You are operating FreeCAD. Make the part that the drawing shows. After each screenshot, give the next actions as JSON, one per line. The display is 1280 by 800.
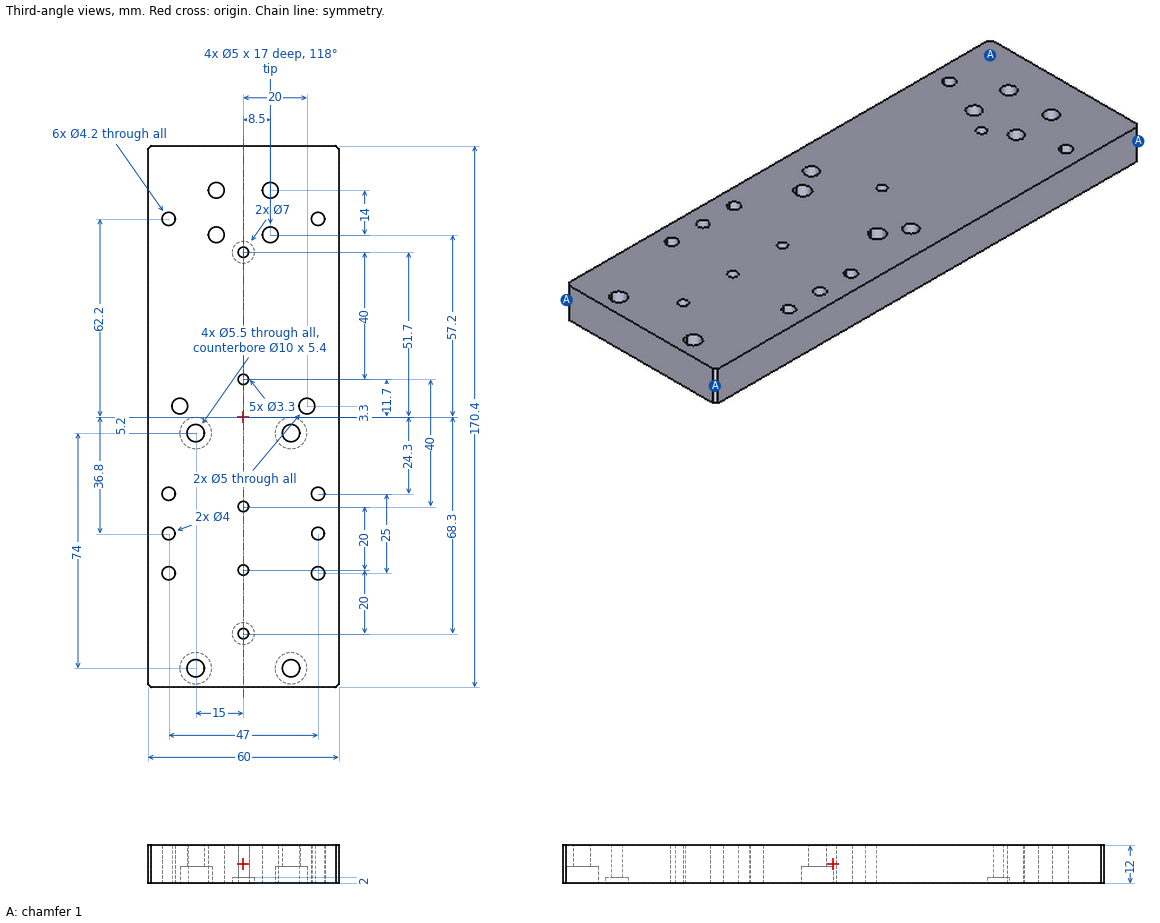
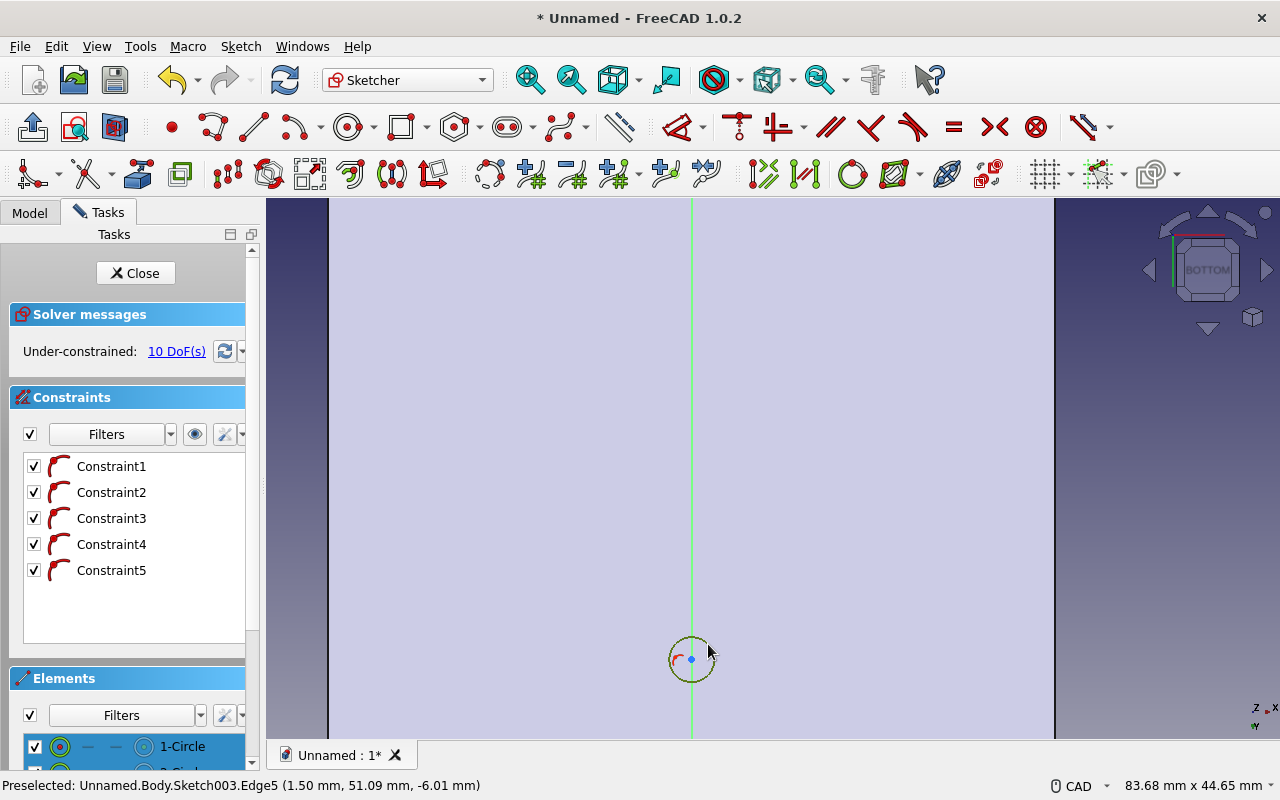
{"action": "left_click", "coordinate": [954, 128]}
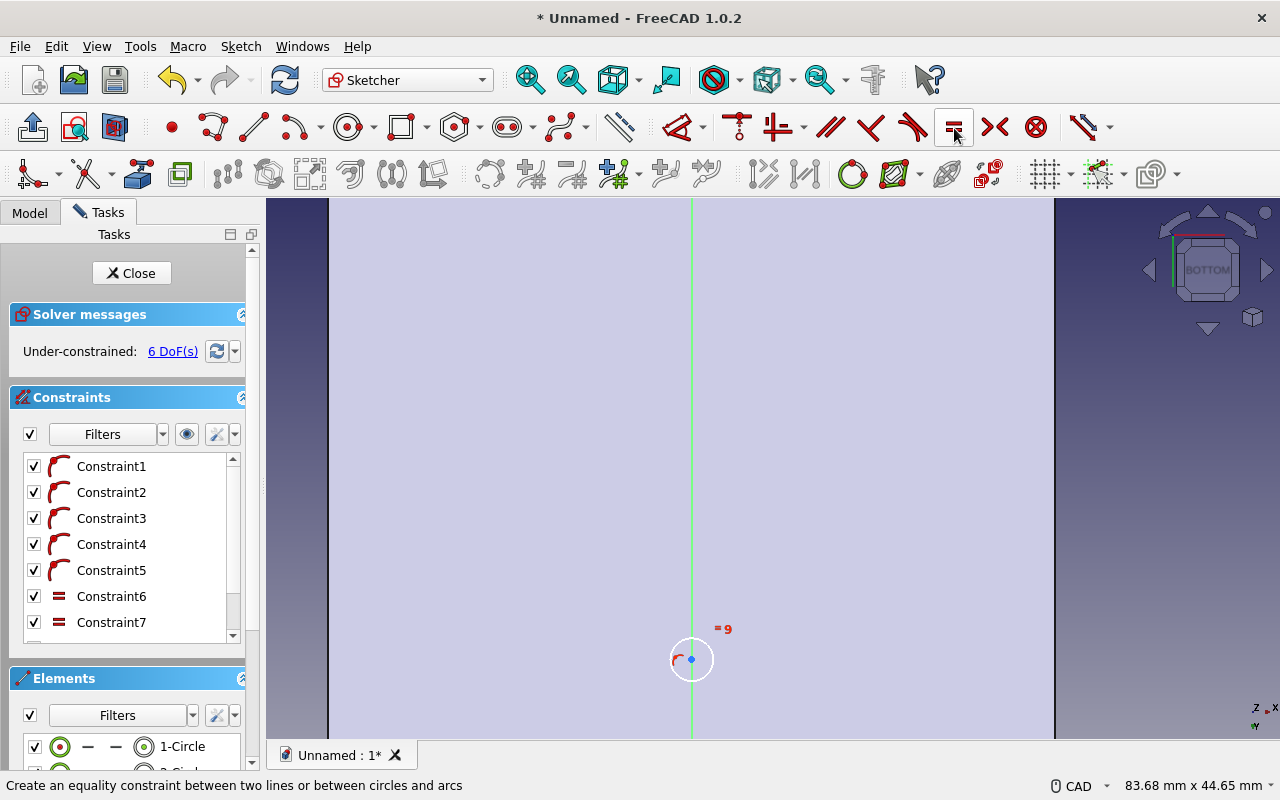
{"action": "left_click", "coordinate": [676, 128]}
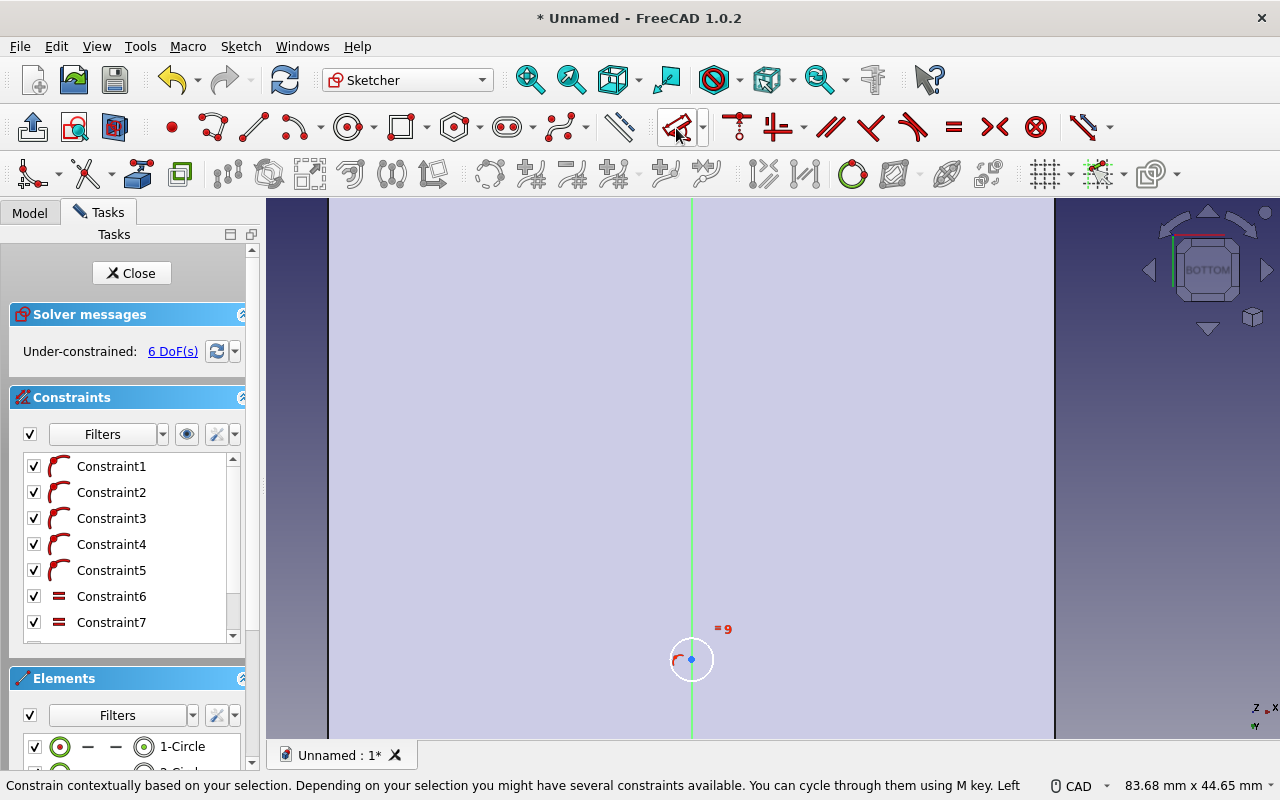
{"action": "scroll", "coordinate": [709, 646], "scroll_direction": "down", "scroll_amount": 7}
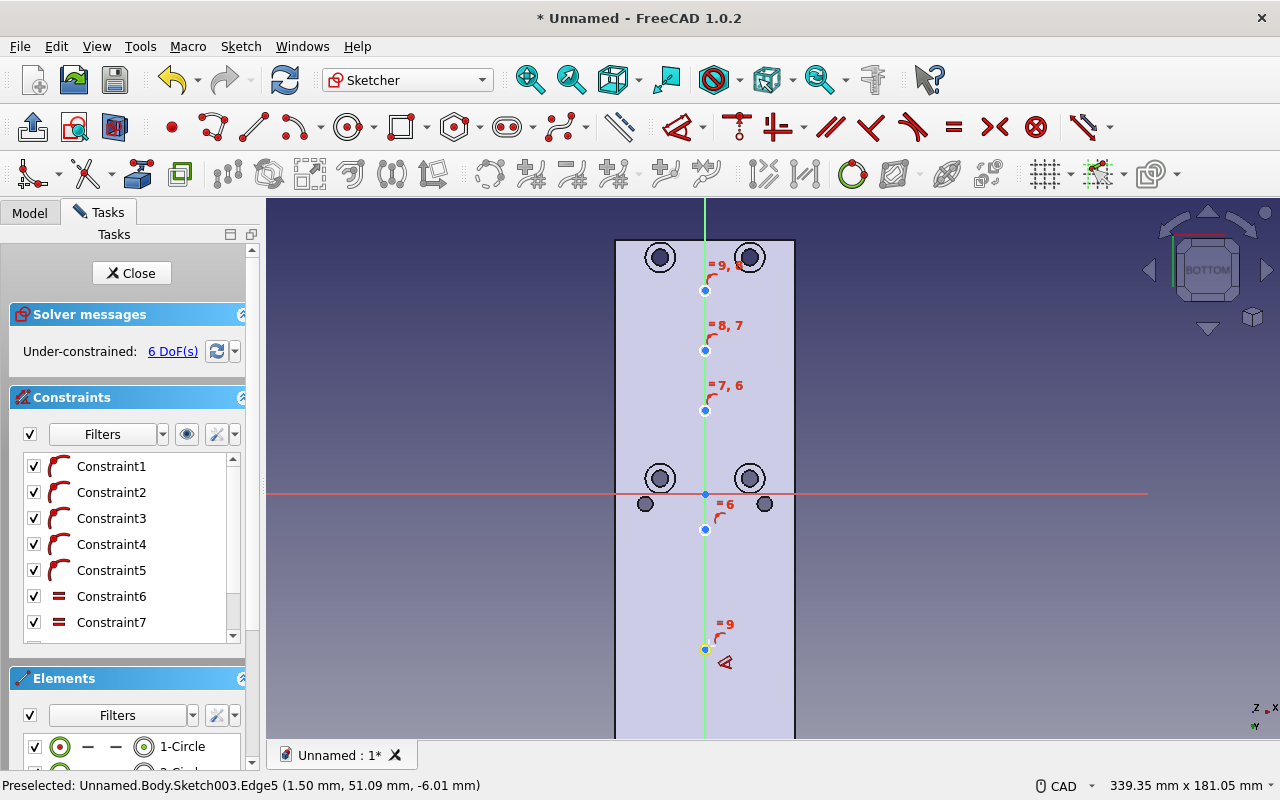
{"action": "scroll", "coordinate": [709, 526], "scroll_direction": "up", "scroll_amount": 7}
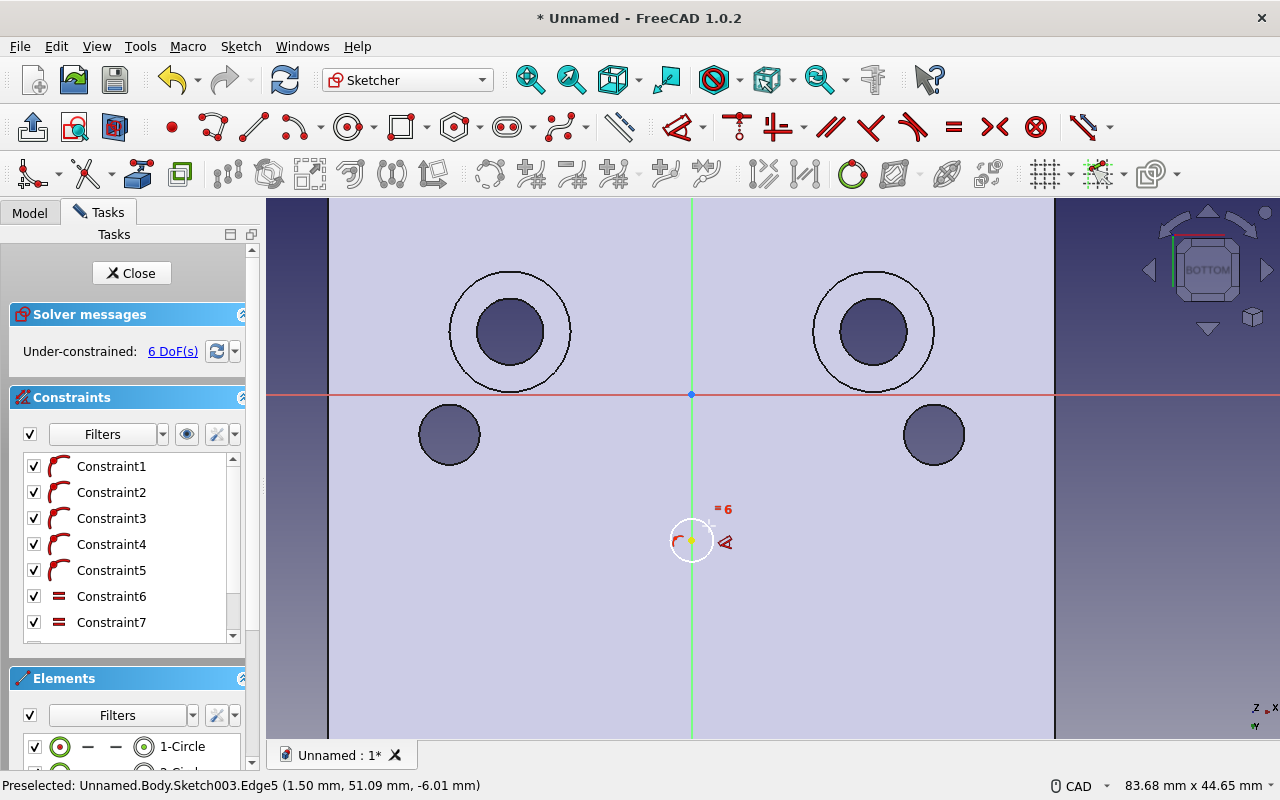
{"action": "left_click", "coordinate": [707, 525]}
{"action": "left_click", "coordinate": [729, 502]}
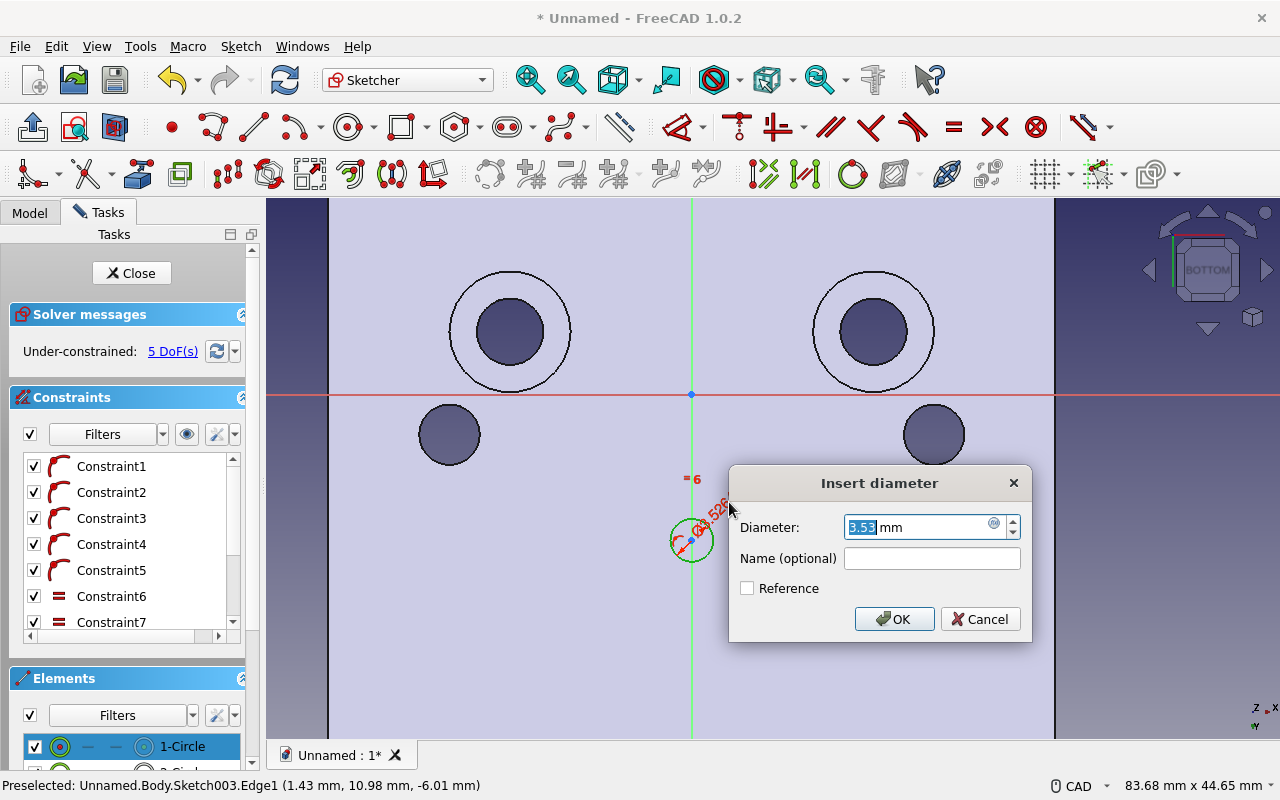
{"action": "type", "text": "3.3"}
{"action": "key", "text": "Return"}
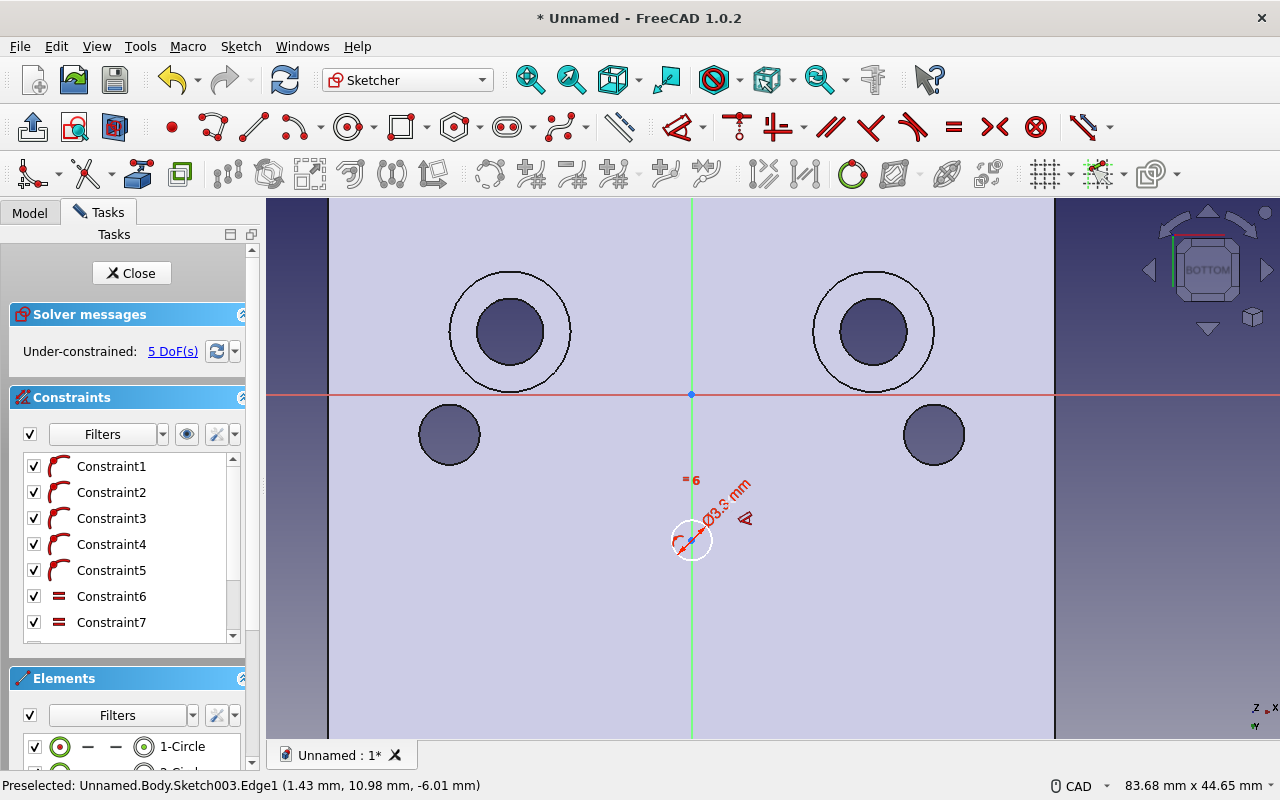
{"action": "scroll", "coordinate": [709, 526], "scroll_direction": "down", "scroll_amount": 7}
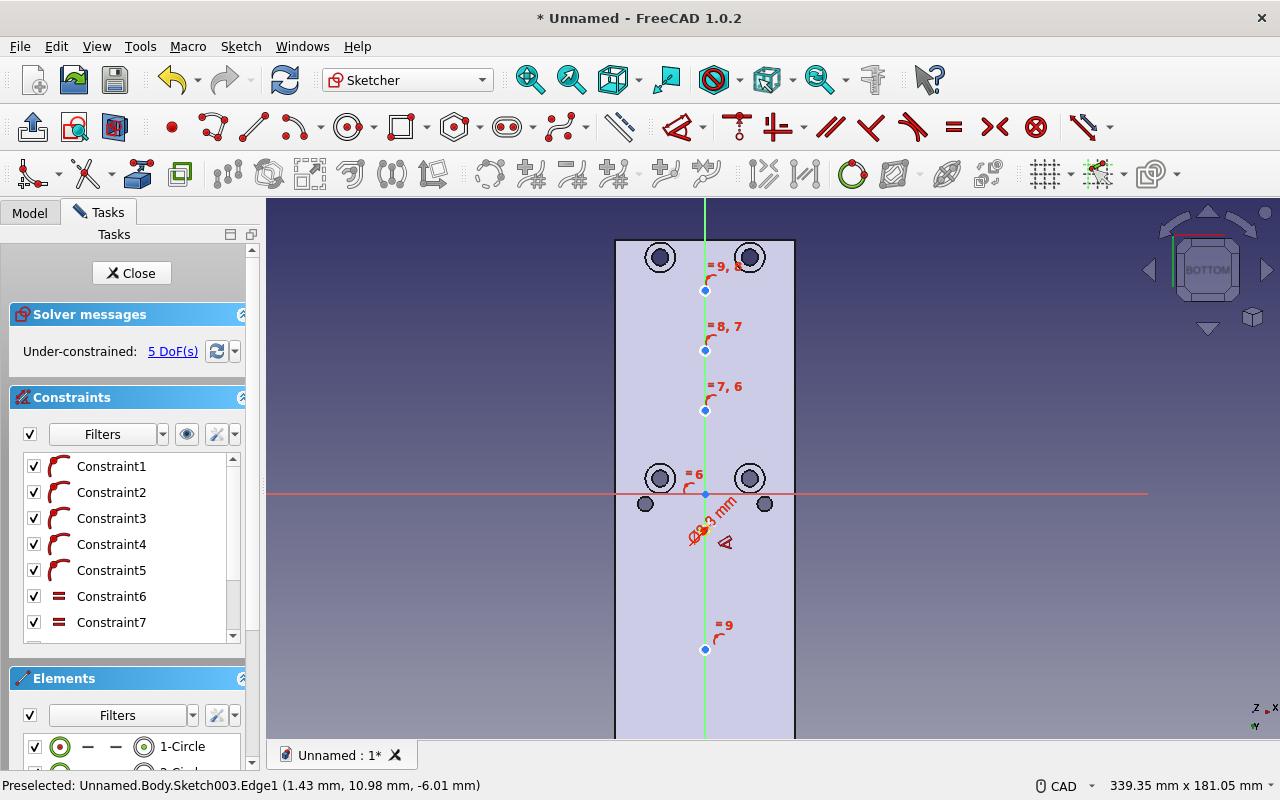
{"action": "left_click", "coordinate": [705, 530]}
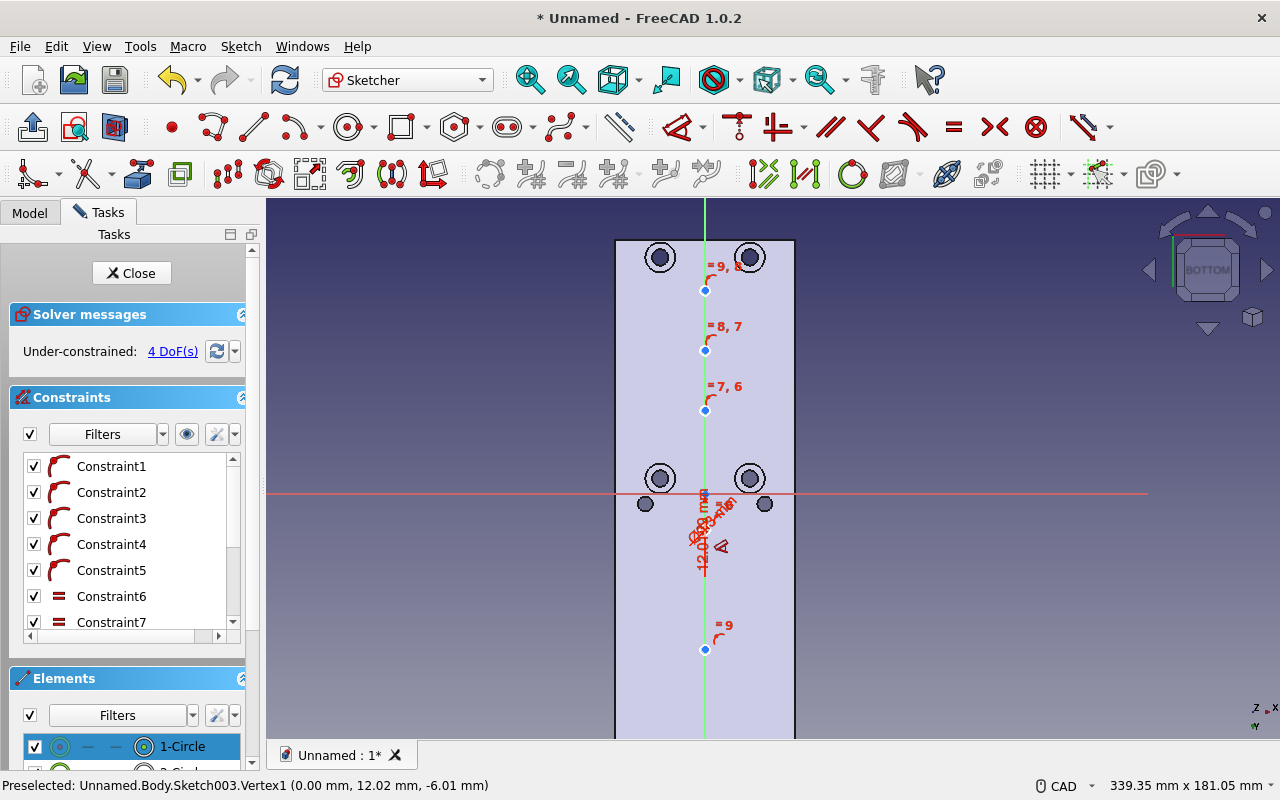
{"action": "left_click", "coordinate": [705, 411]}
{"action": "left_click", "coordinate": [739, 470]}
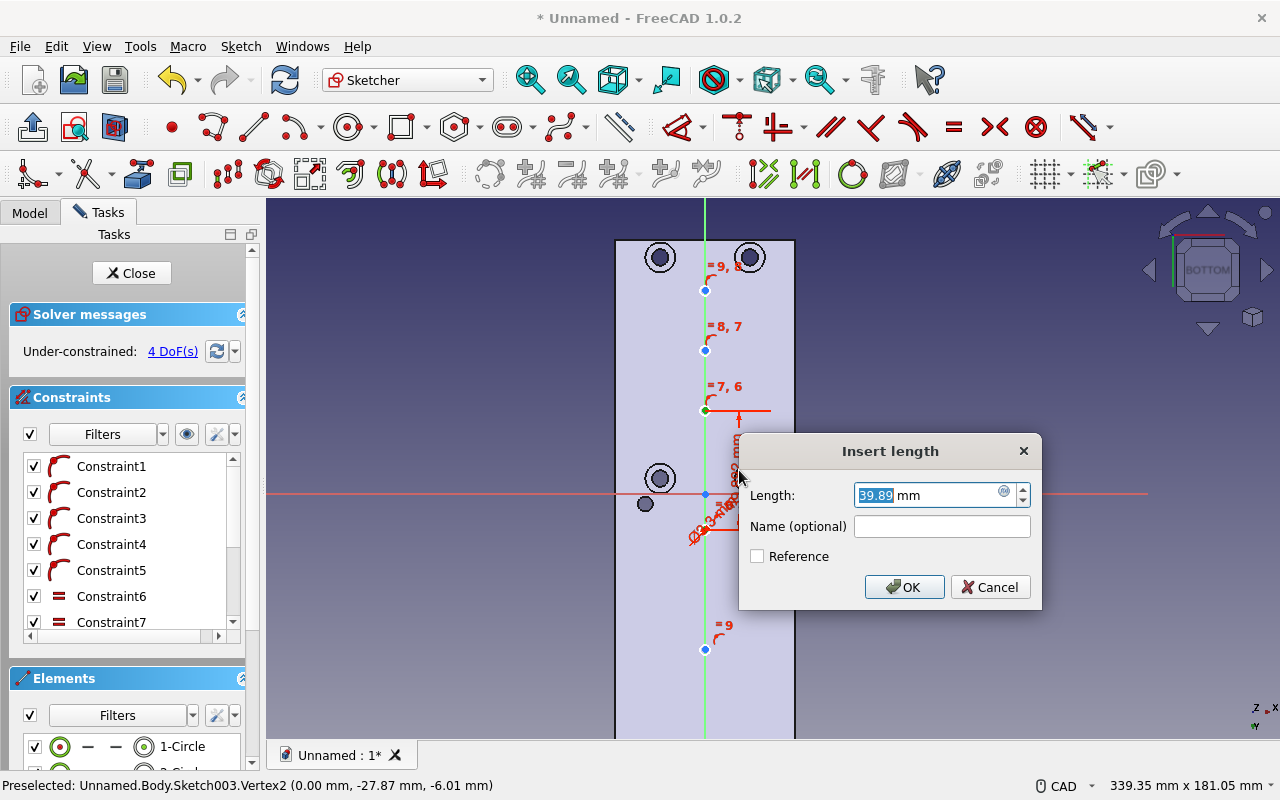
{"action": "type", "text": "40"}
{"action": "key", "text": "Return"}